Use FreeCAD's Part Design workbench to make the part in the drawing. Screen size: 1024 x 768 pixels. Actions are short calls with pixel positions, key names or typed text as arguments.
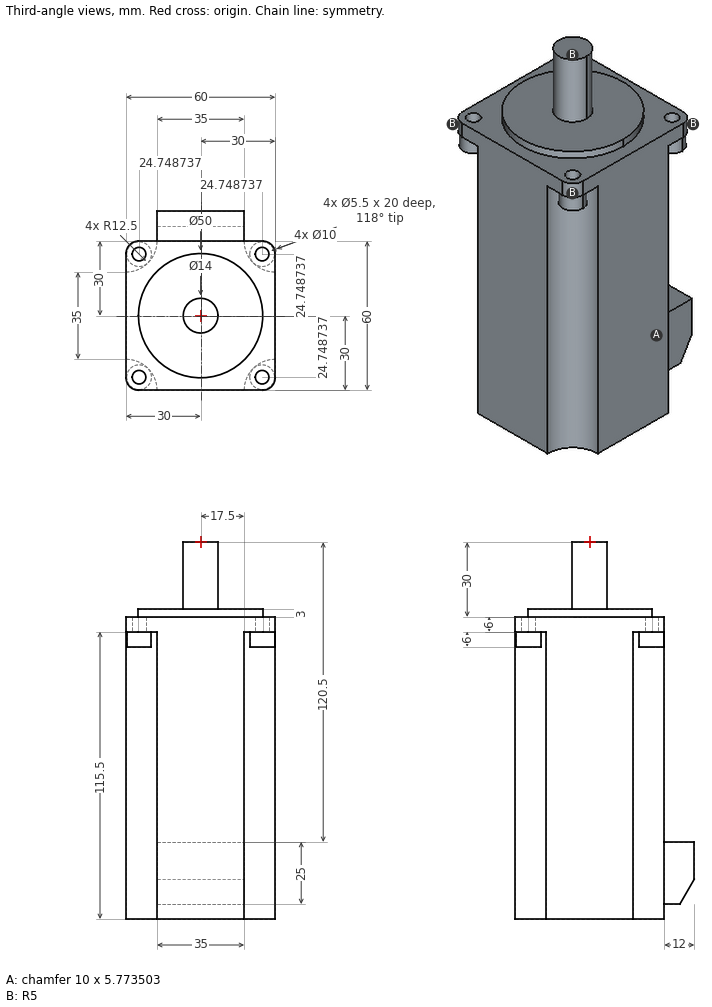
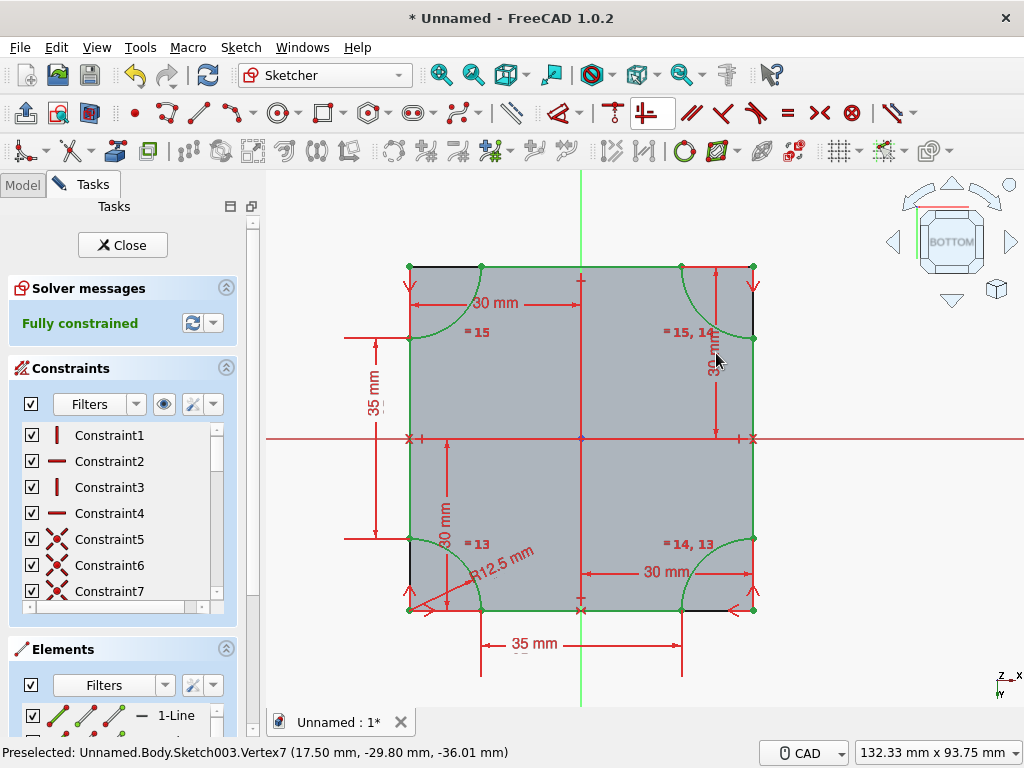
click(123, 245)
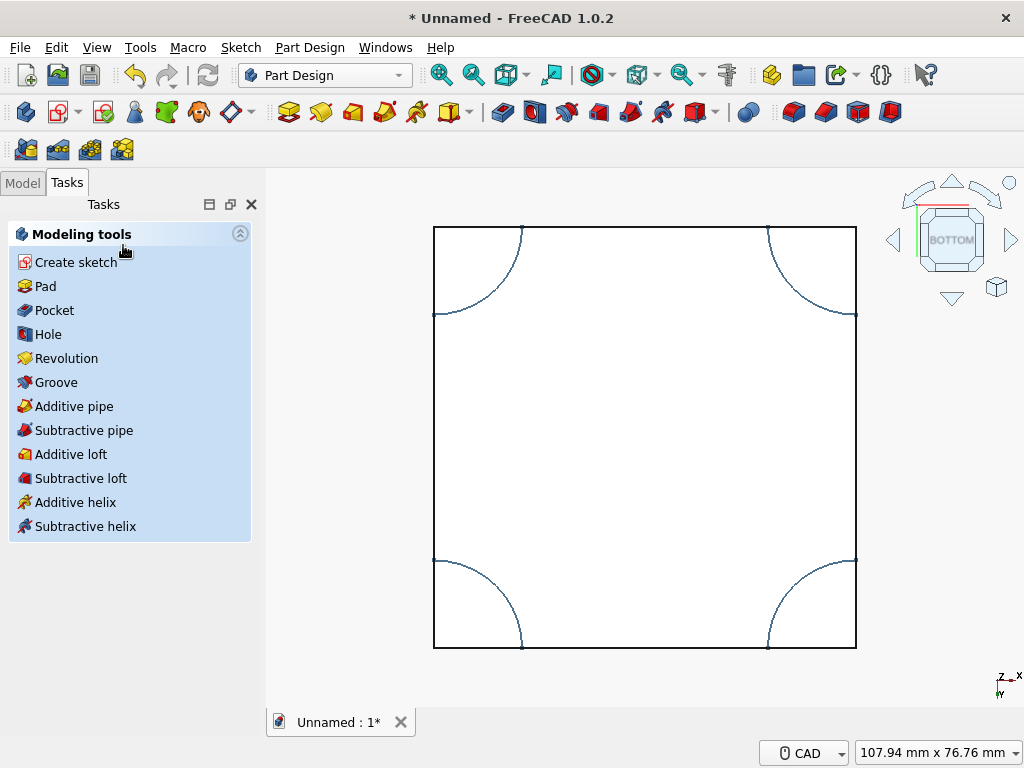
click(290, 112)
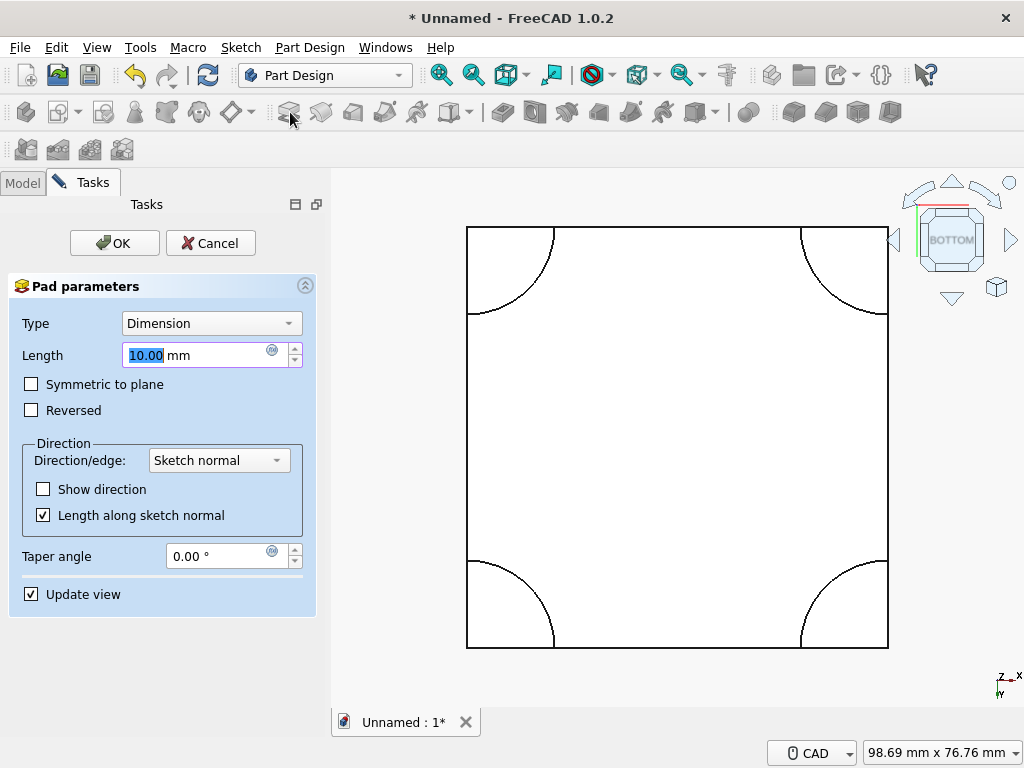
text(115.5)
key(Tab)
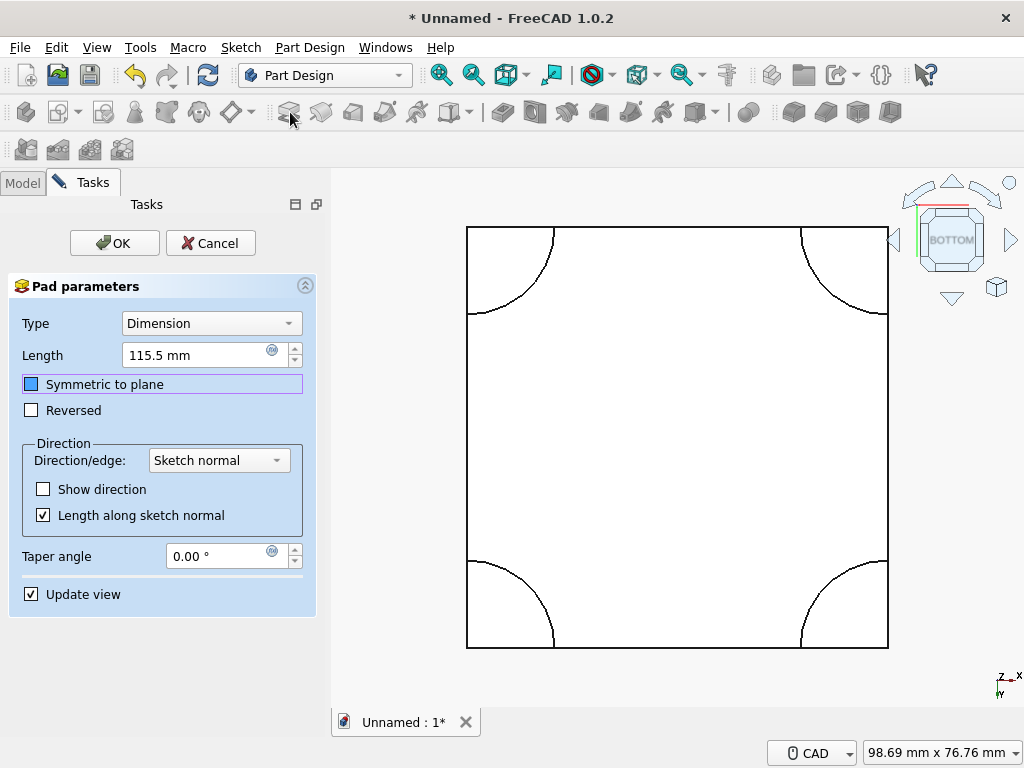
click(115, 243)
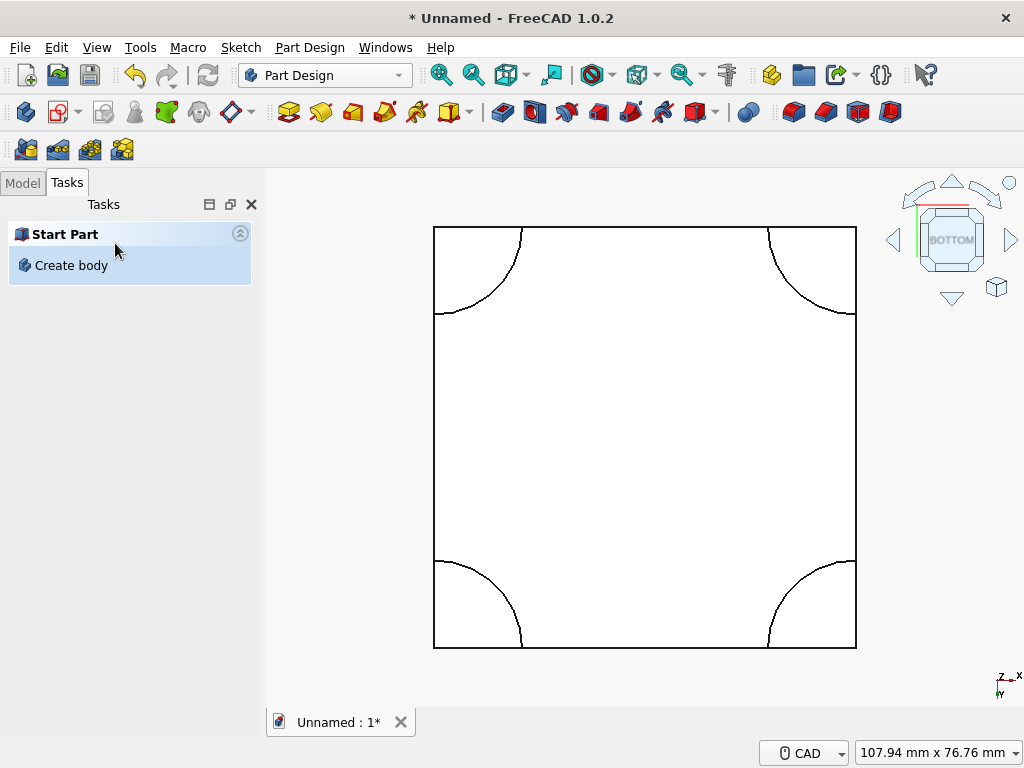
key(4)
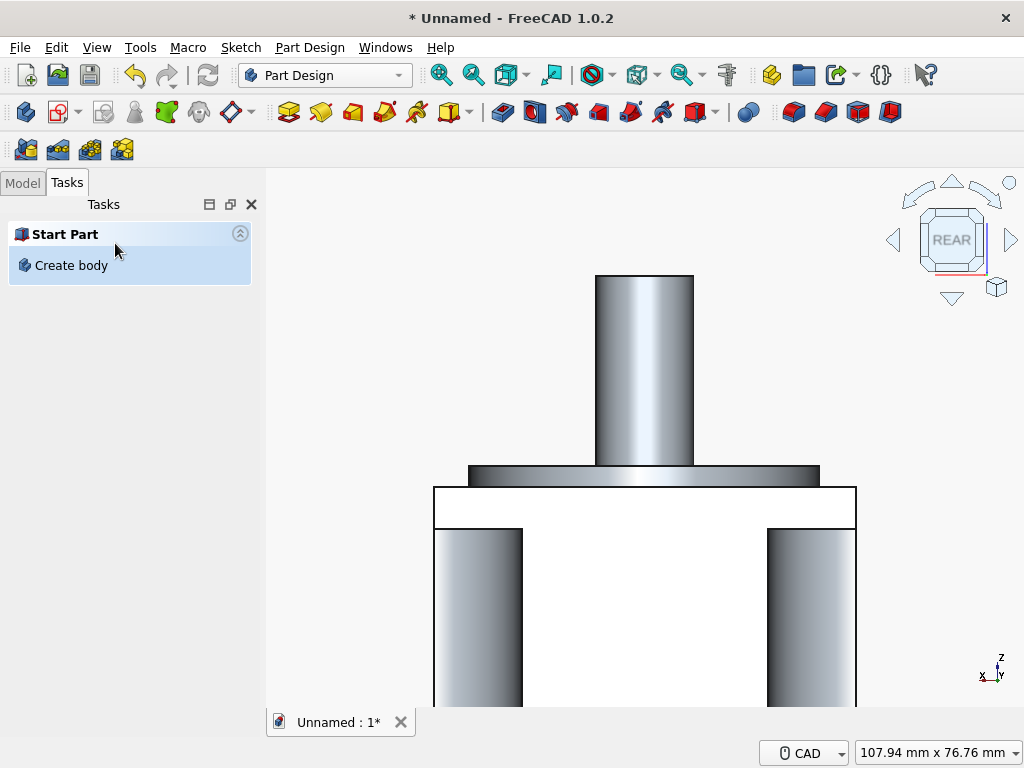
click(442, 76)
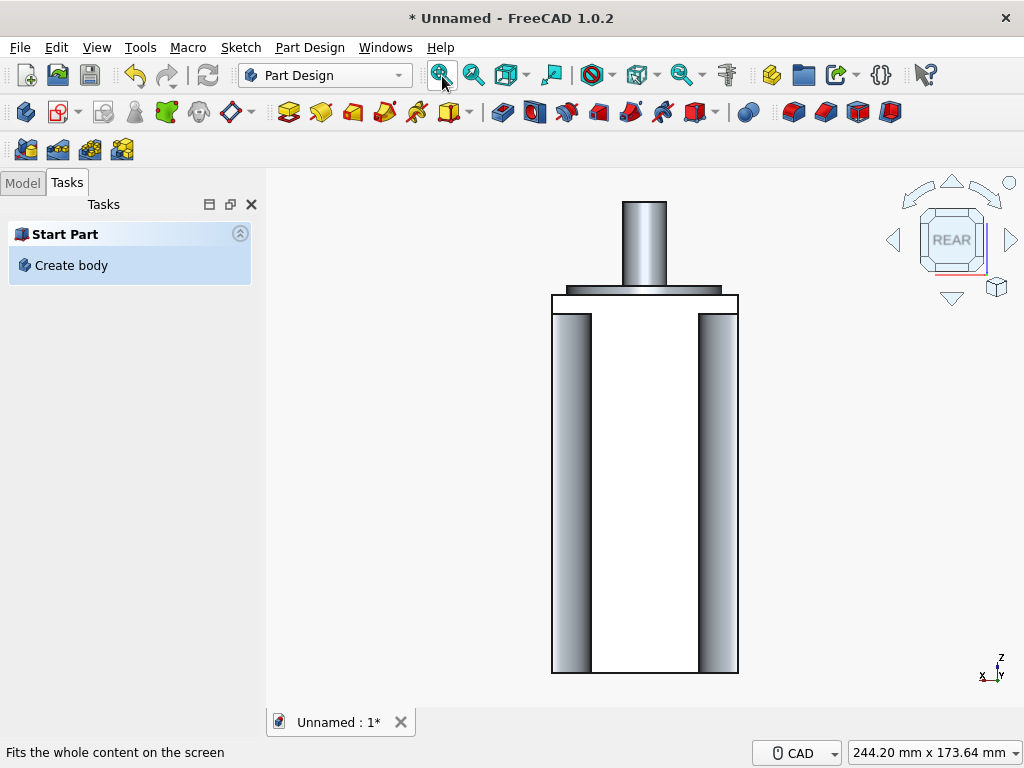
click(645, 375)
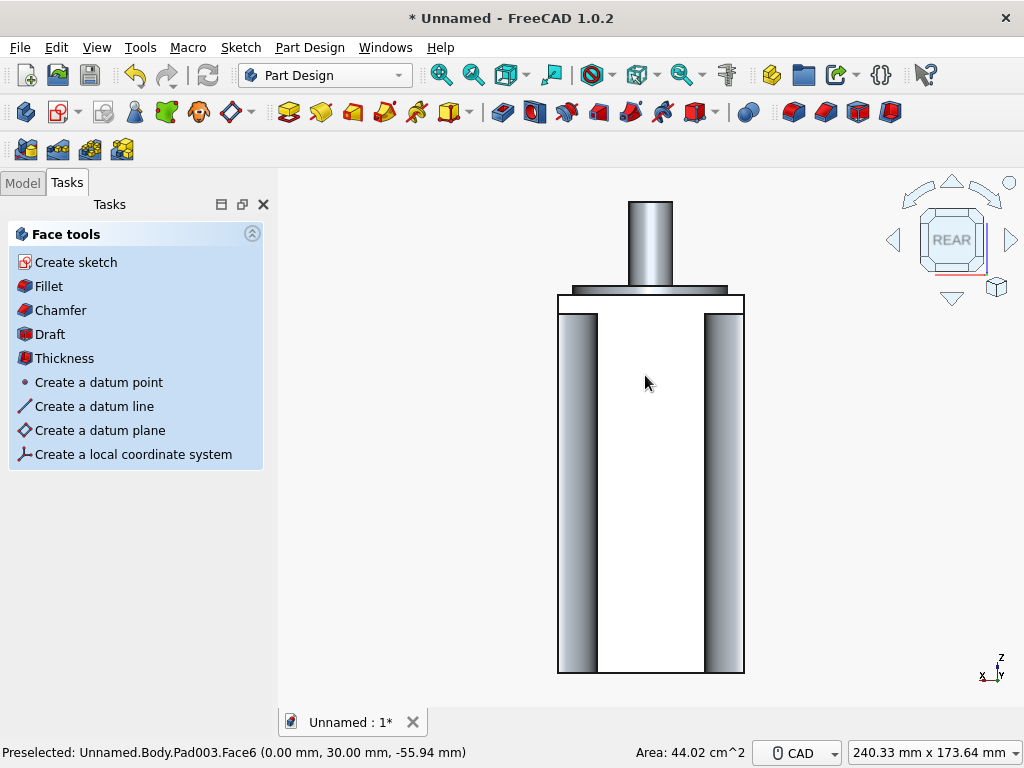
click(58, 112)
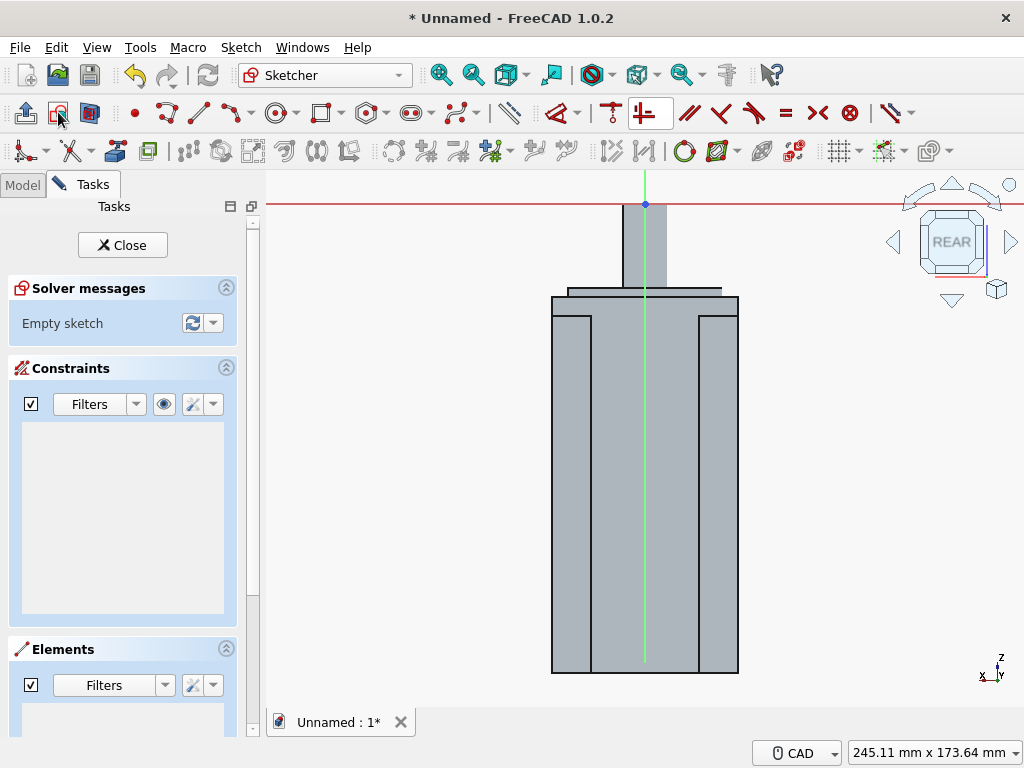
scroll(667, 673, up, 7)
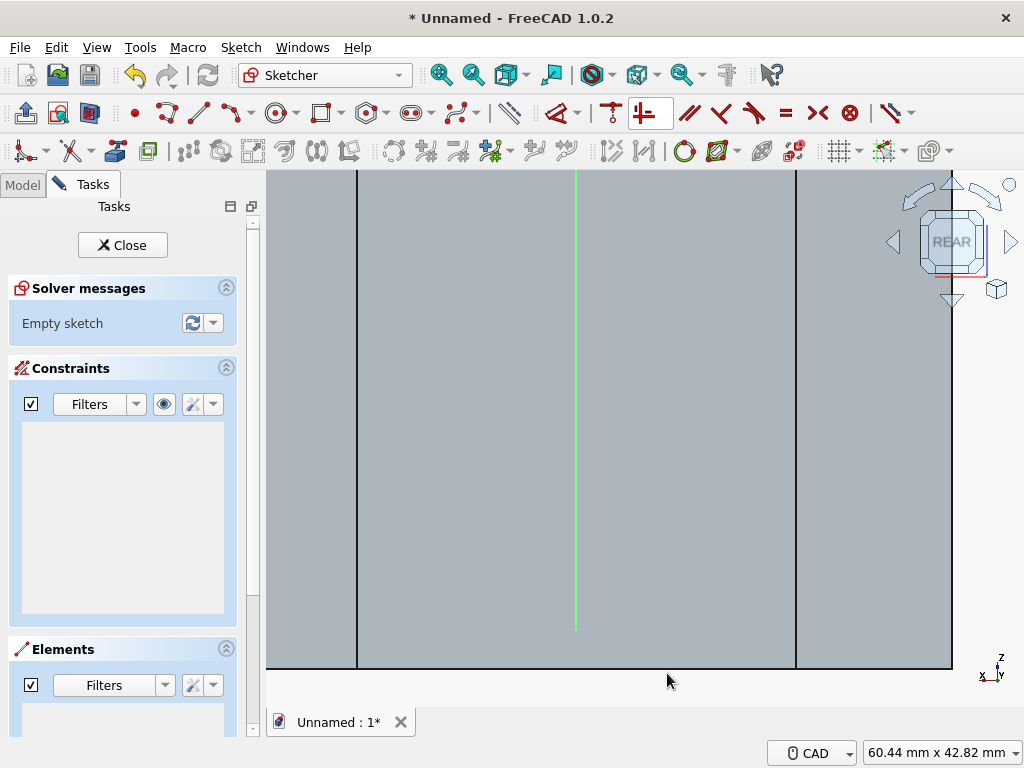
click(322, 114)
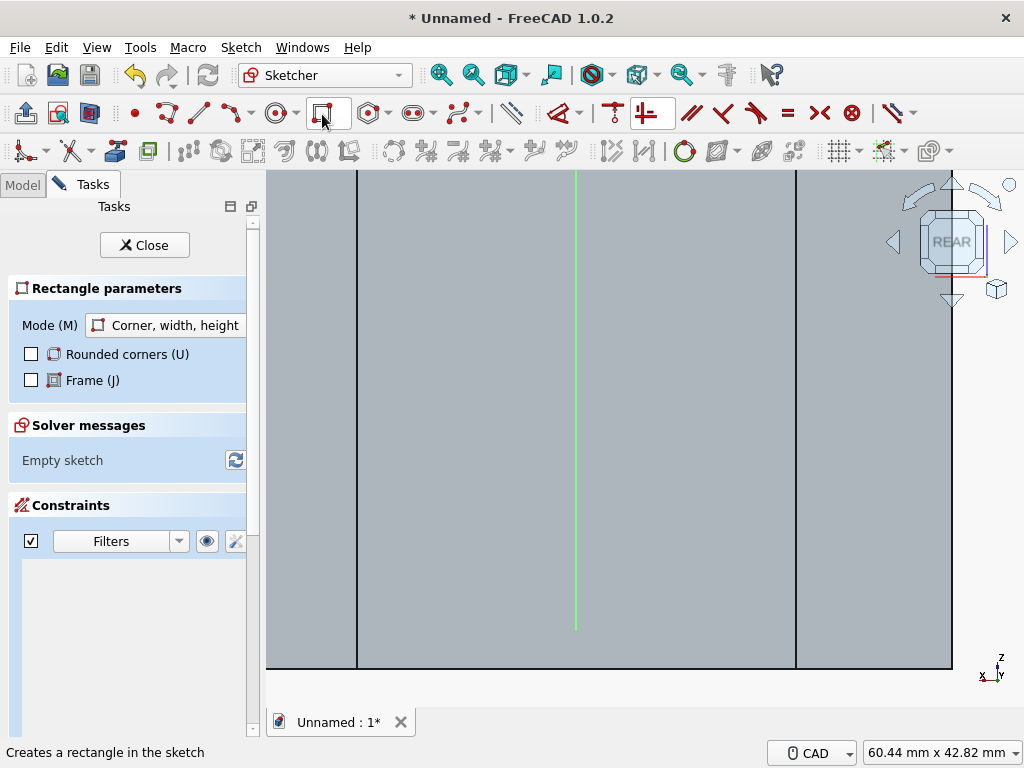
click(357, 280)
click(796, 594)
key(Escape)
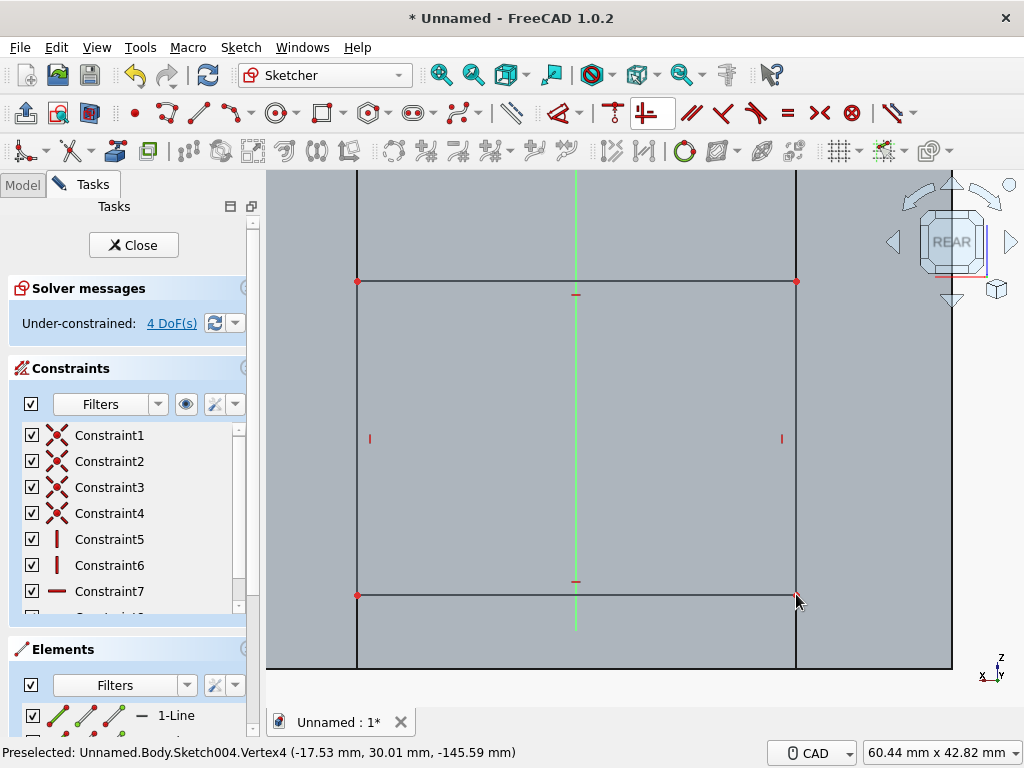
click(558, 114)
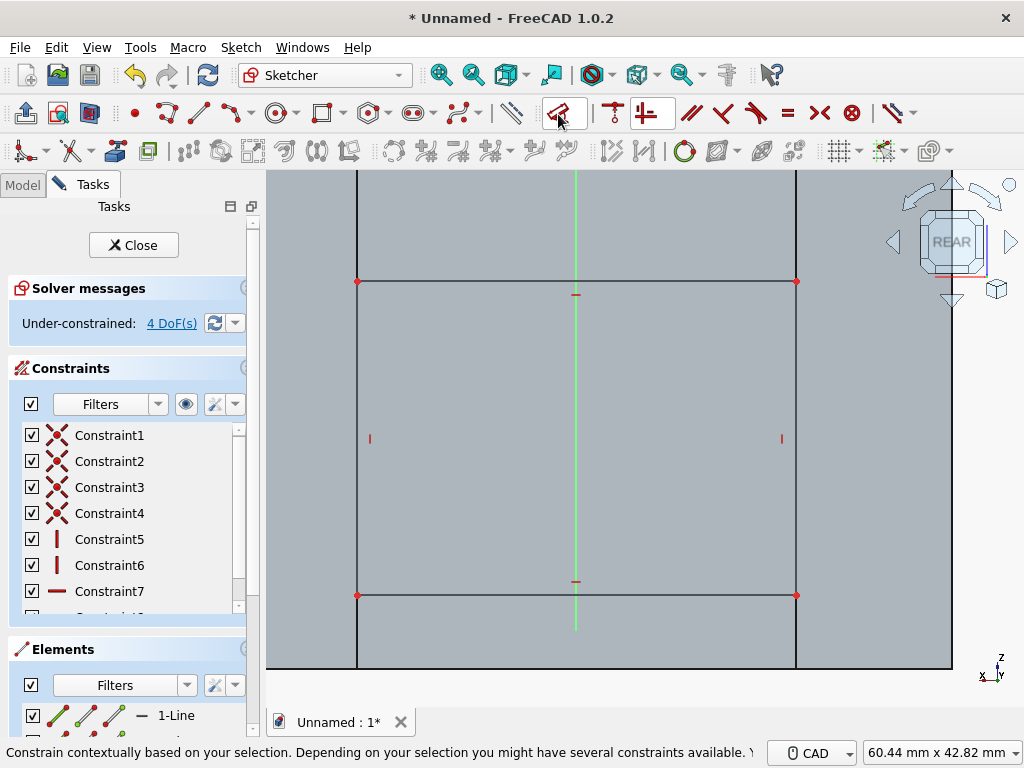
click(357, 375)
click(323, 438)